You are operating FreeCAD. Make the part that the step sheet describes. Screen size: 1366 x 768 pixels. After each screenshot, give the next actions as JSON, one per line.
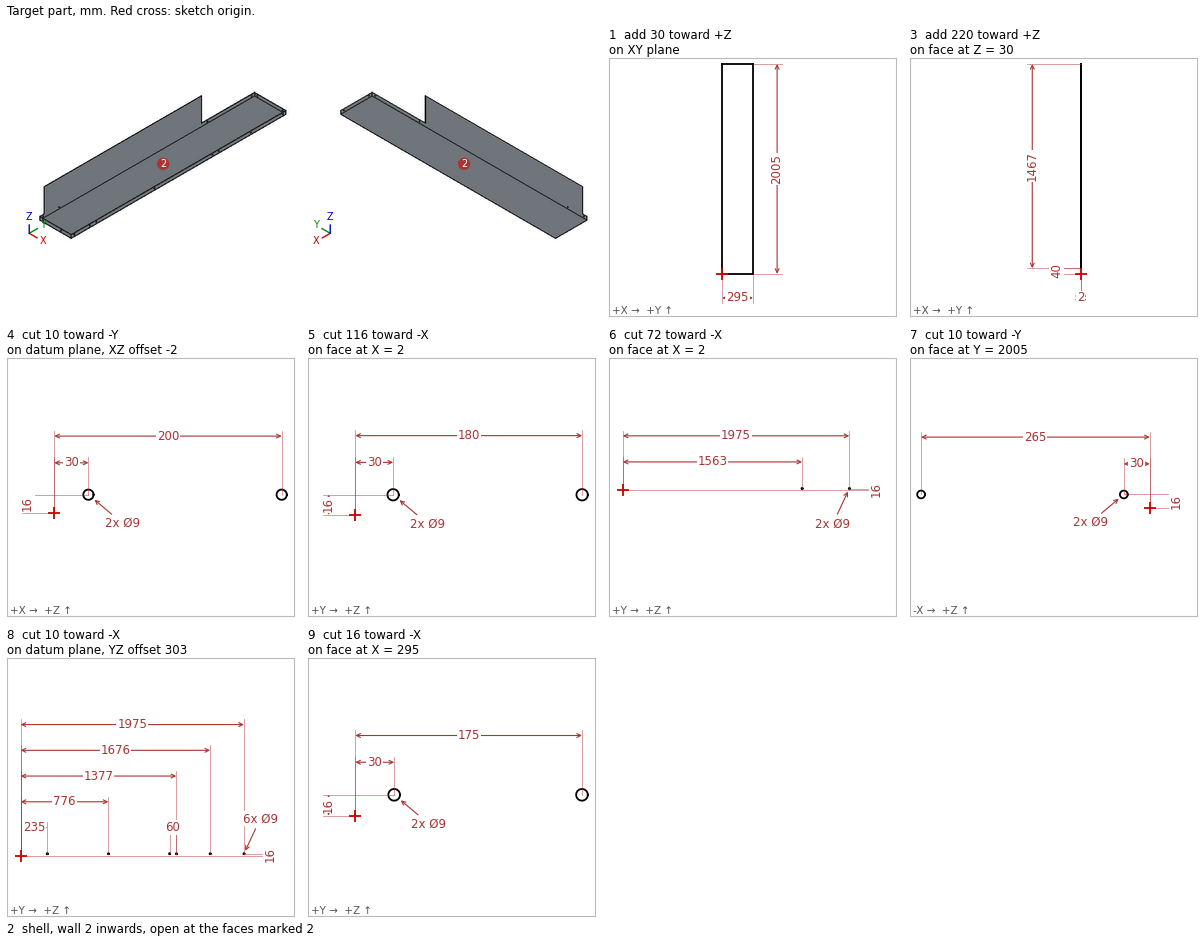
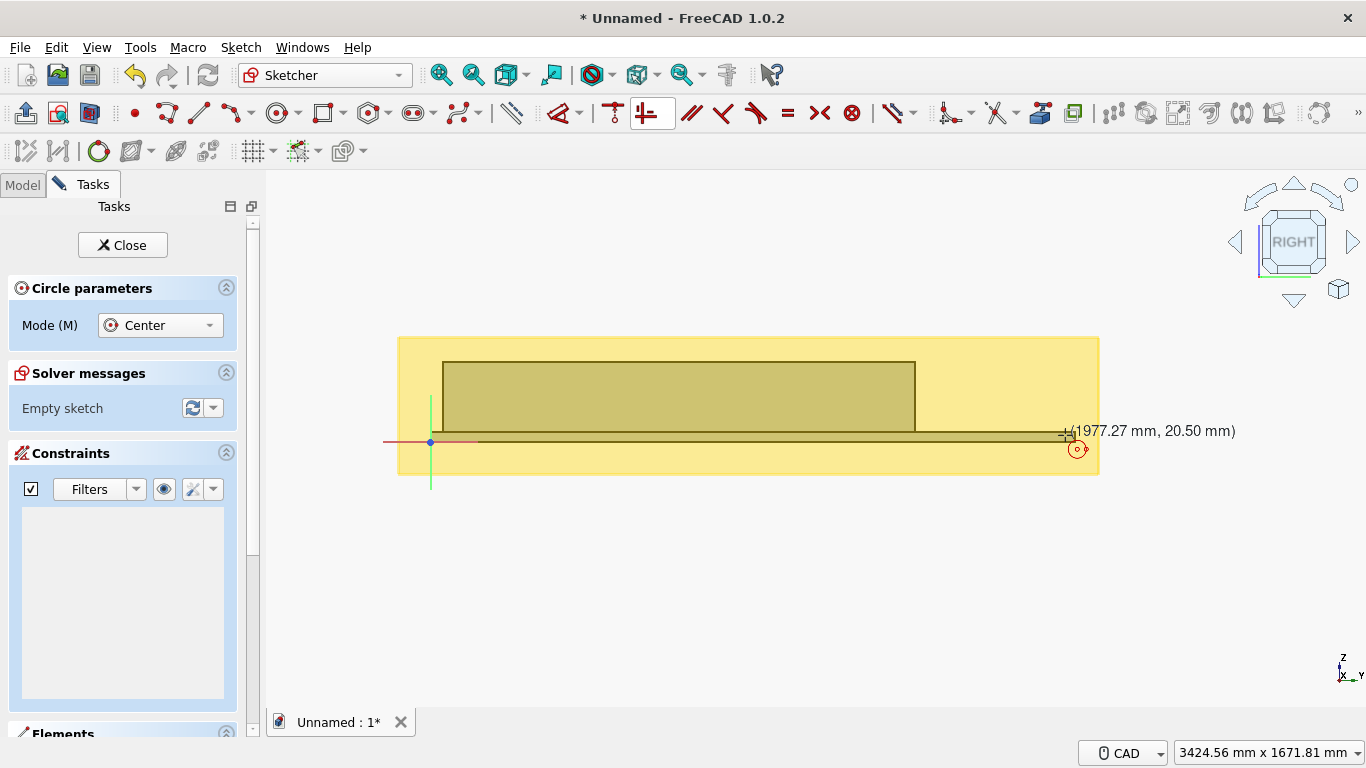
{"action": "scroll", "coordinate": [1065, 437], "scroll_direction": "up", "scroll_amount": 6}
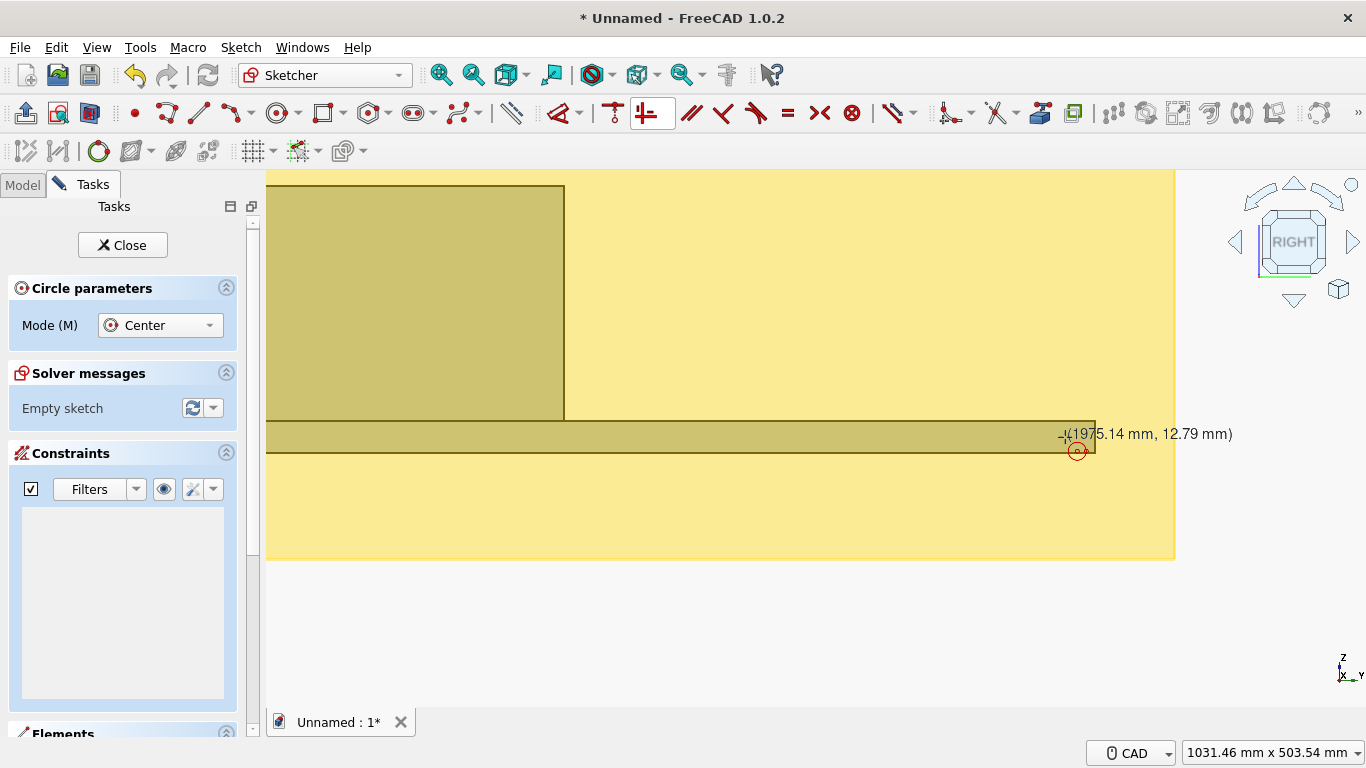
{"action": "left_click", "coordinate": [1063, 436]}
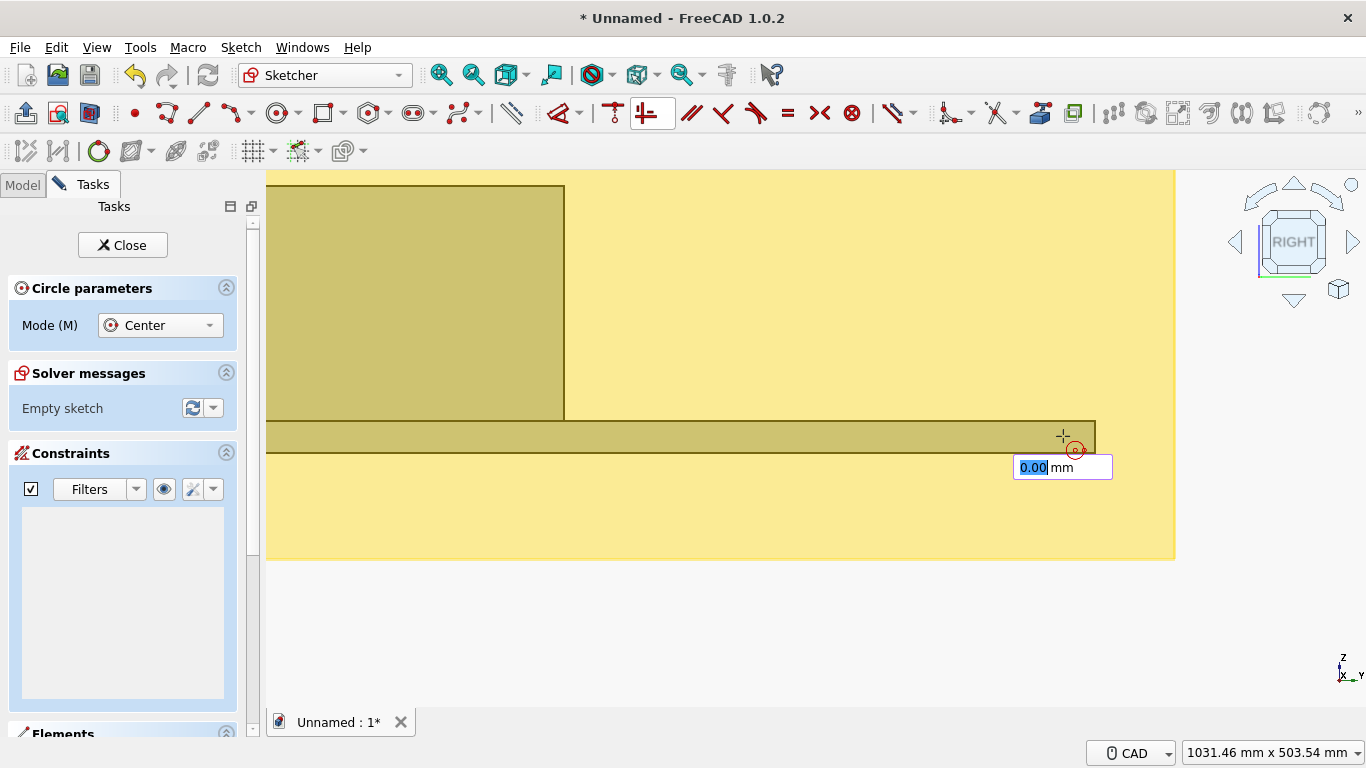
{"action": "scroll", "coordinate": [1067, 432], "scroll_direction": "up", "scroll_amount": 6}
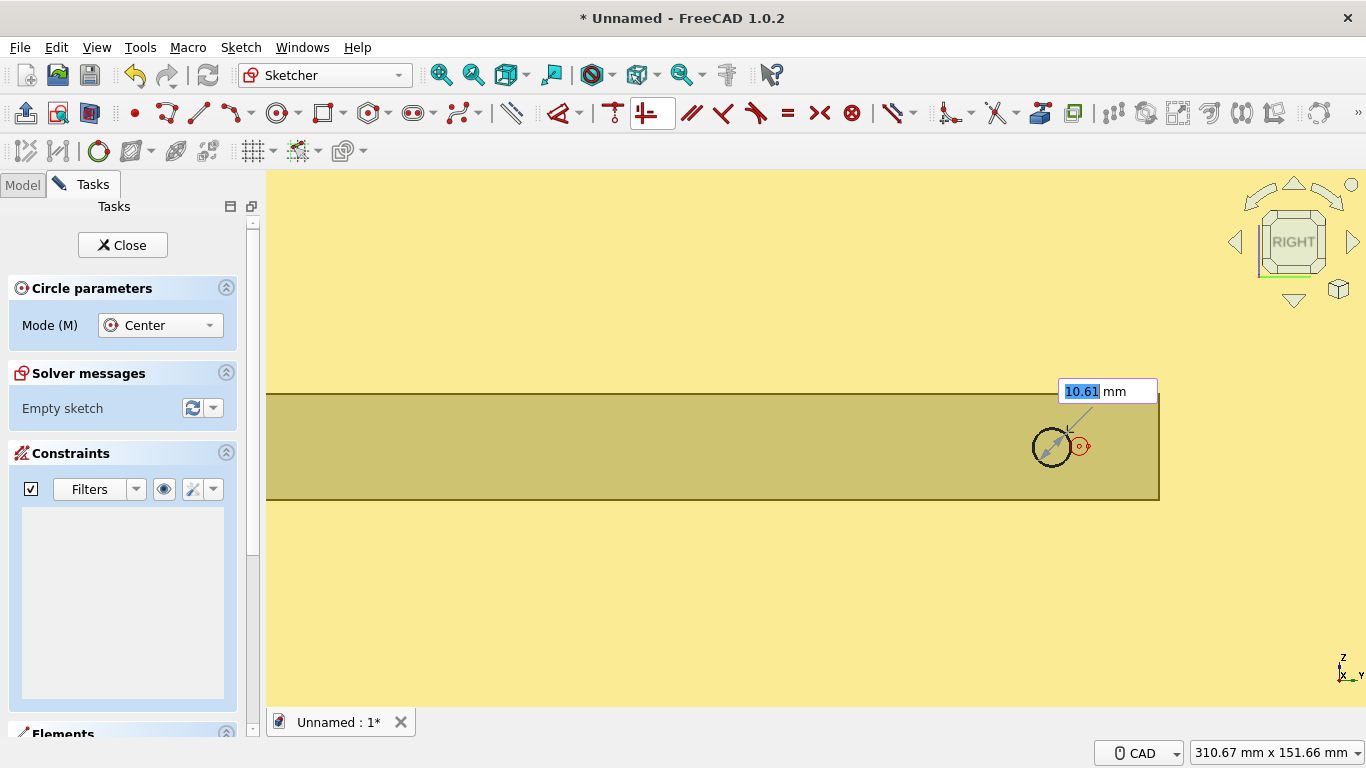
{"action": "left_click", "coordinate": [1064, 432]}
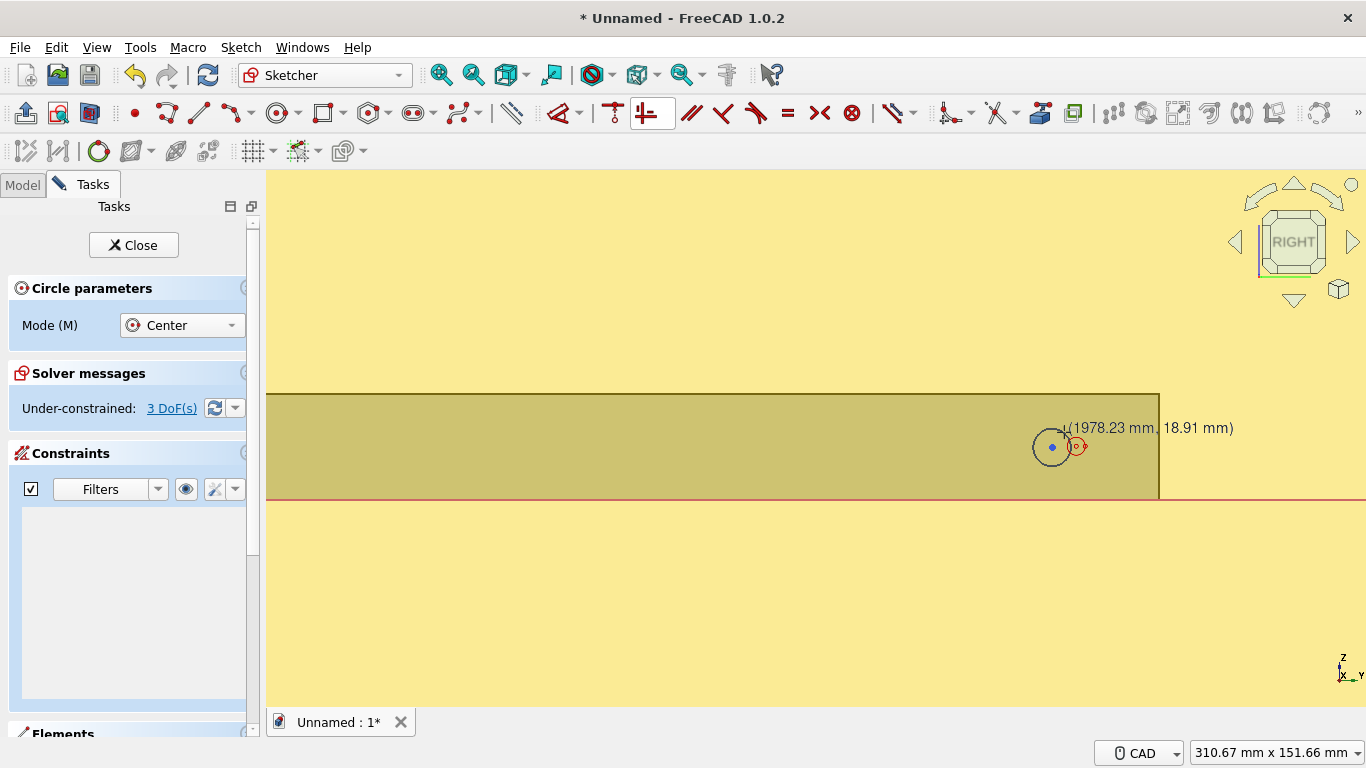
{"action": "scroll", "coordinate": [1065, 436], "scroll_direction": "down", "scroll_amount": 12}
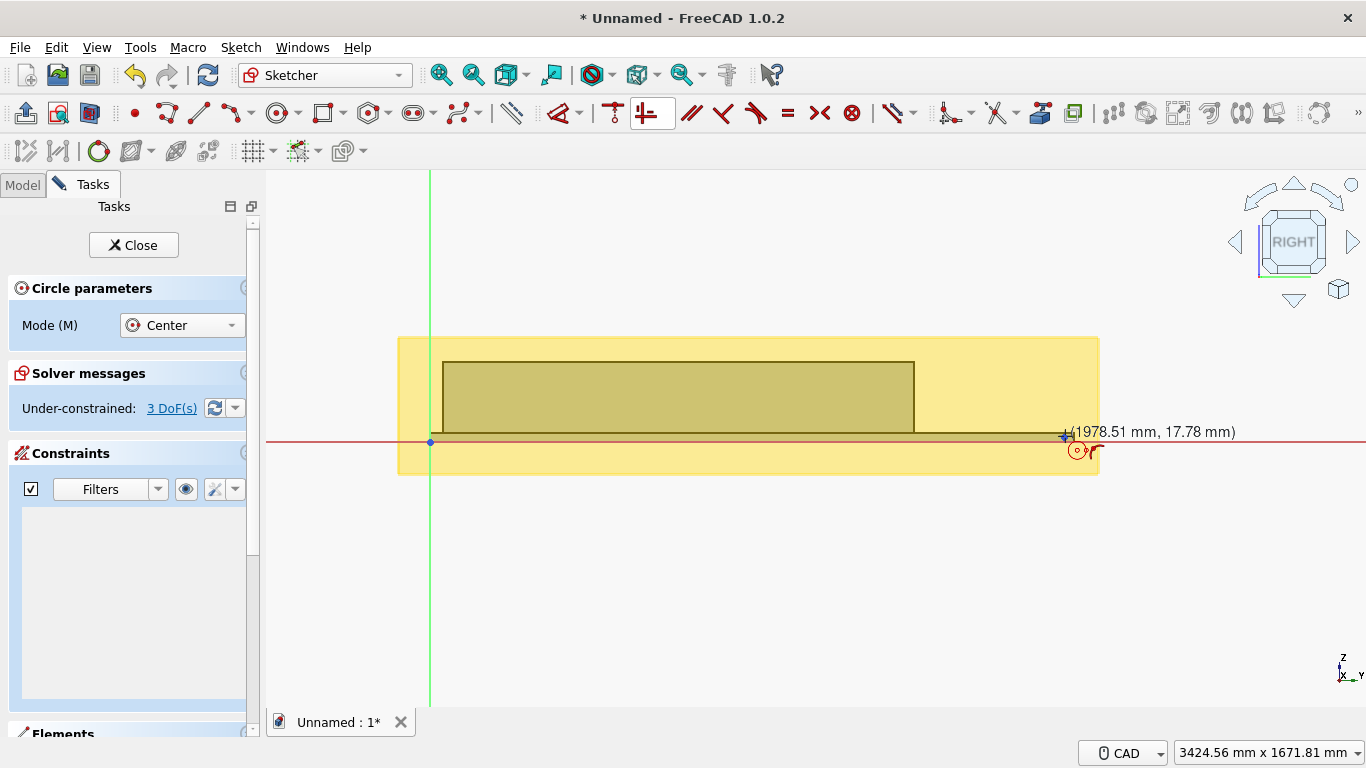
{"action": "scroll", "coordinate": [968, 437], "scroll_direction": "up", "scroll_amount": 14}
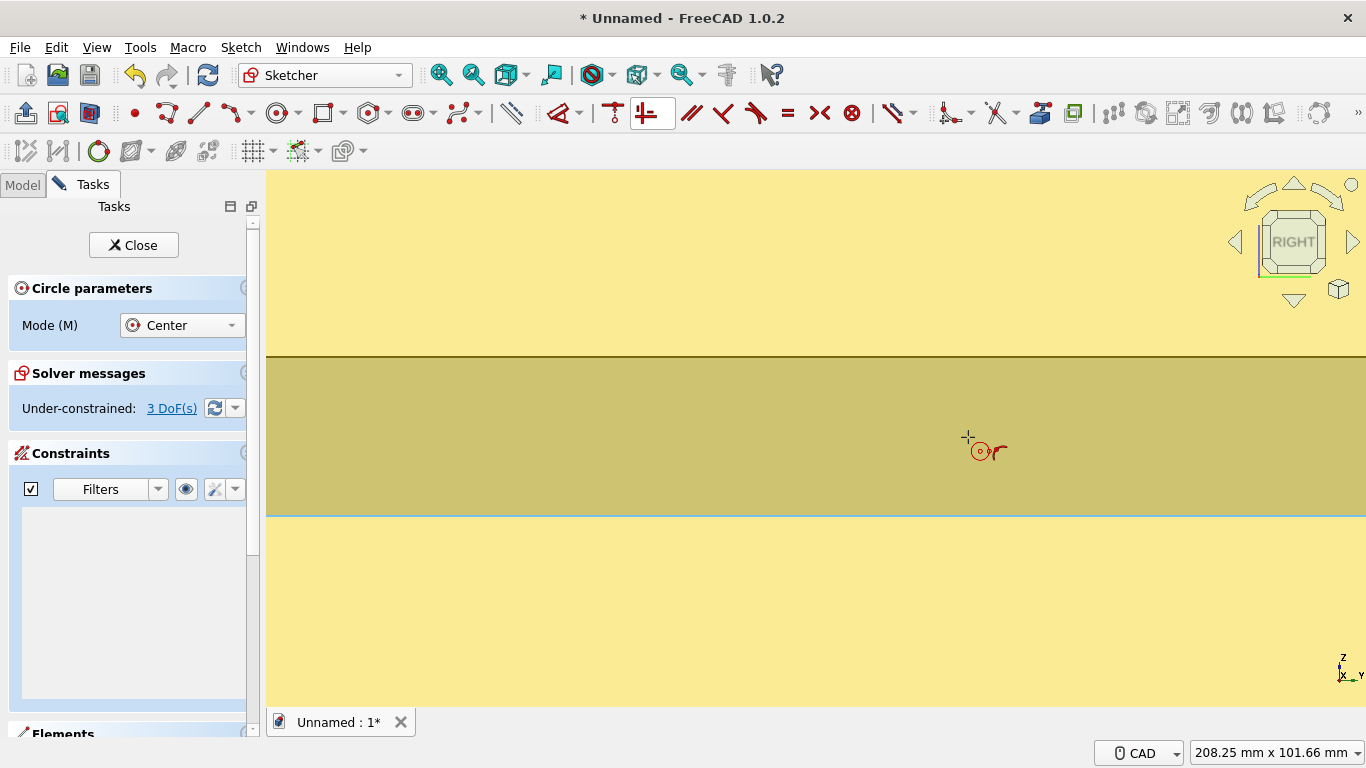
{"action": "scroll", "coordinate": [968, 437], "scroll_direction": "down", "scroll_amount": 14}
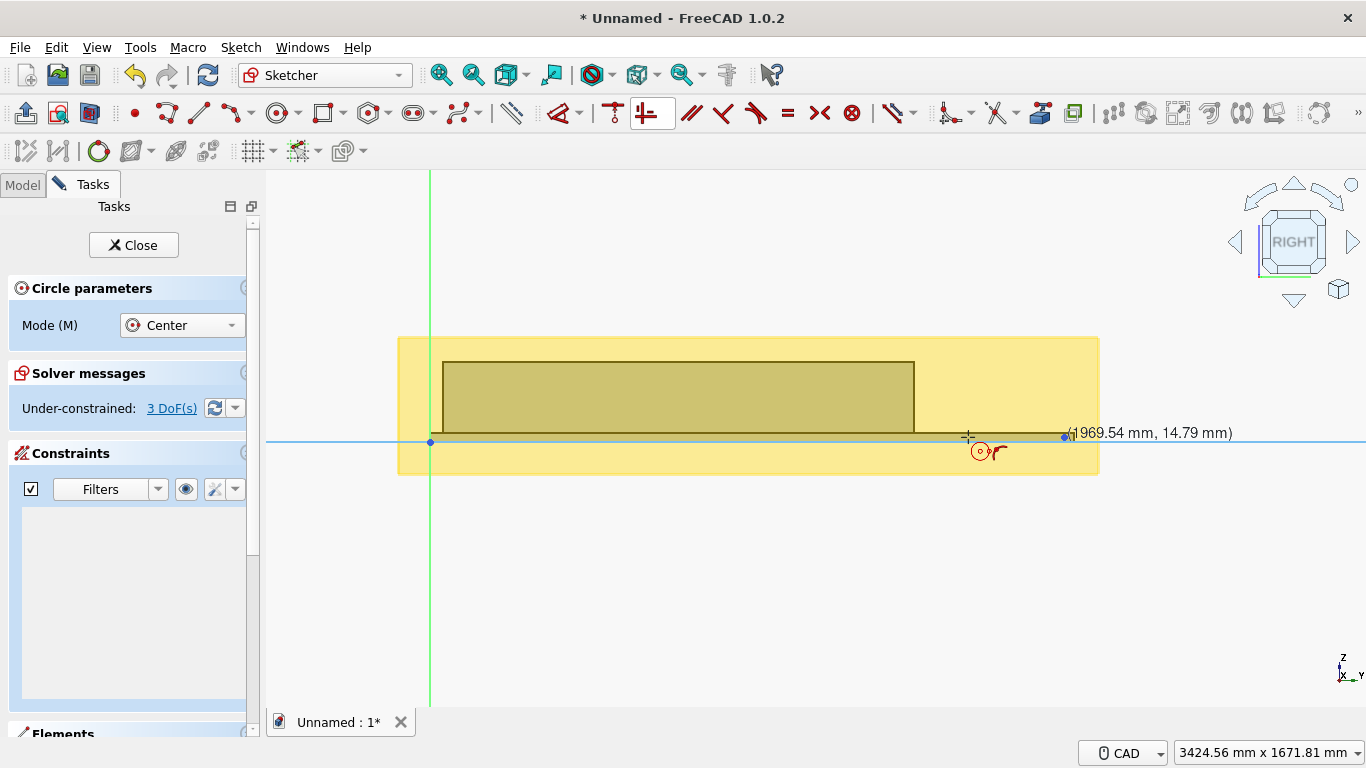
{"action": "scroll", "coordinate": [968, 437], "scroll_direction": "up", "scroll_amount": 6}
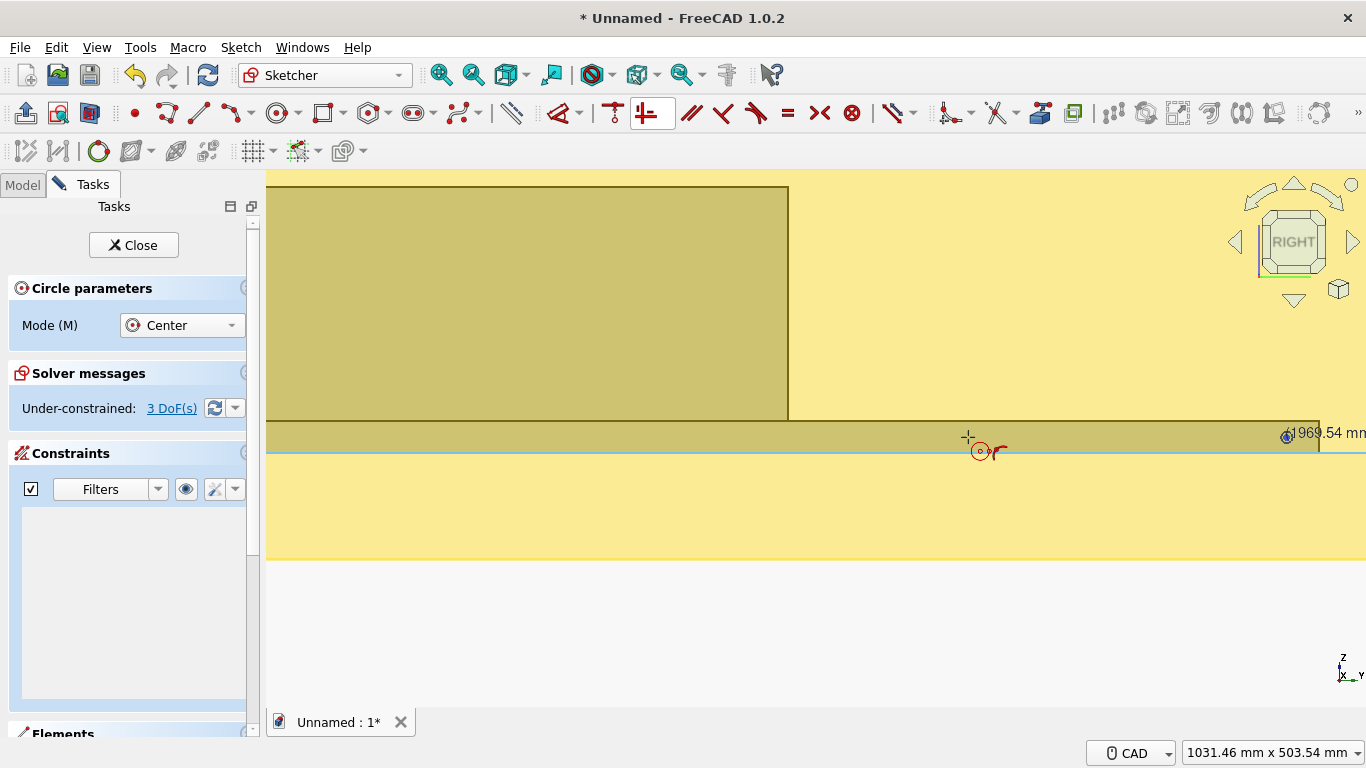
{"action": "left_click", "coordinate": [968, 436]}